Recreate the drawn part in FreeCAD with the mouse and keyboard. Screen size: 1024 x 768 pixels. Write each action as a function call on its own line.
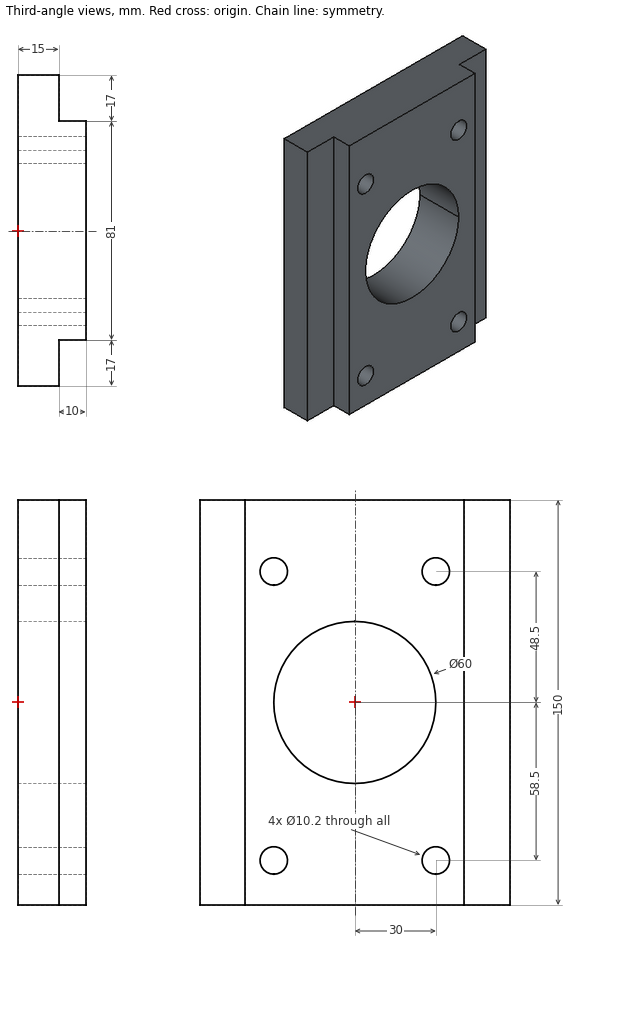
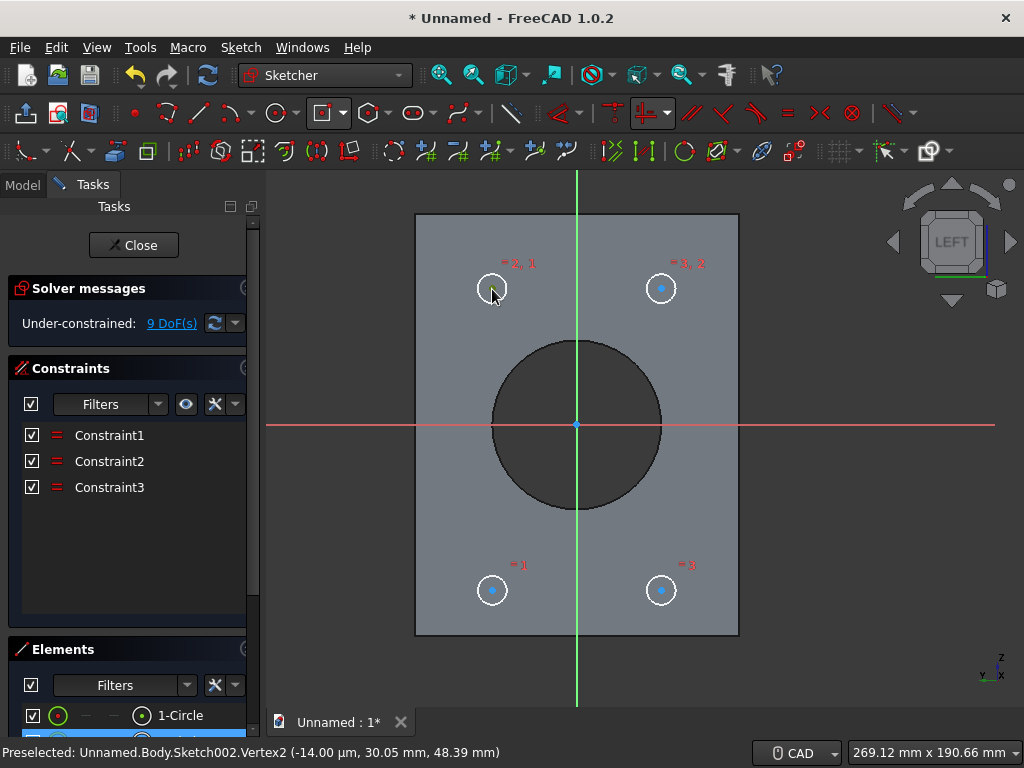
click(661, 289)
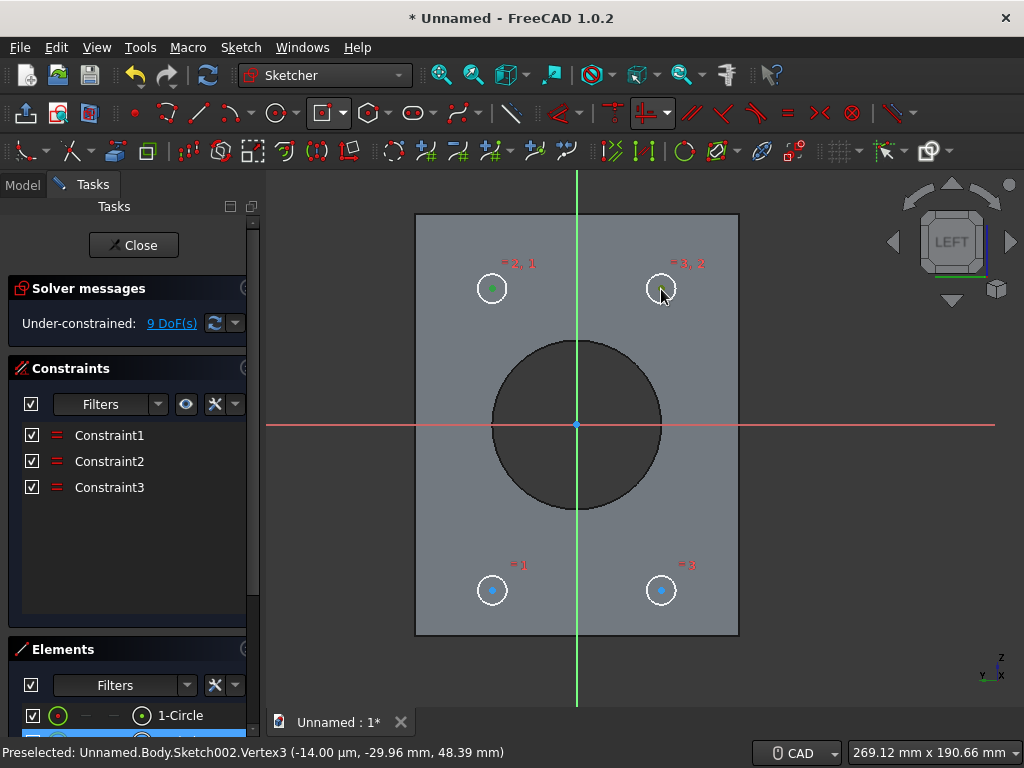
click(577, 645)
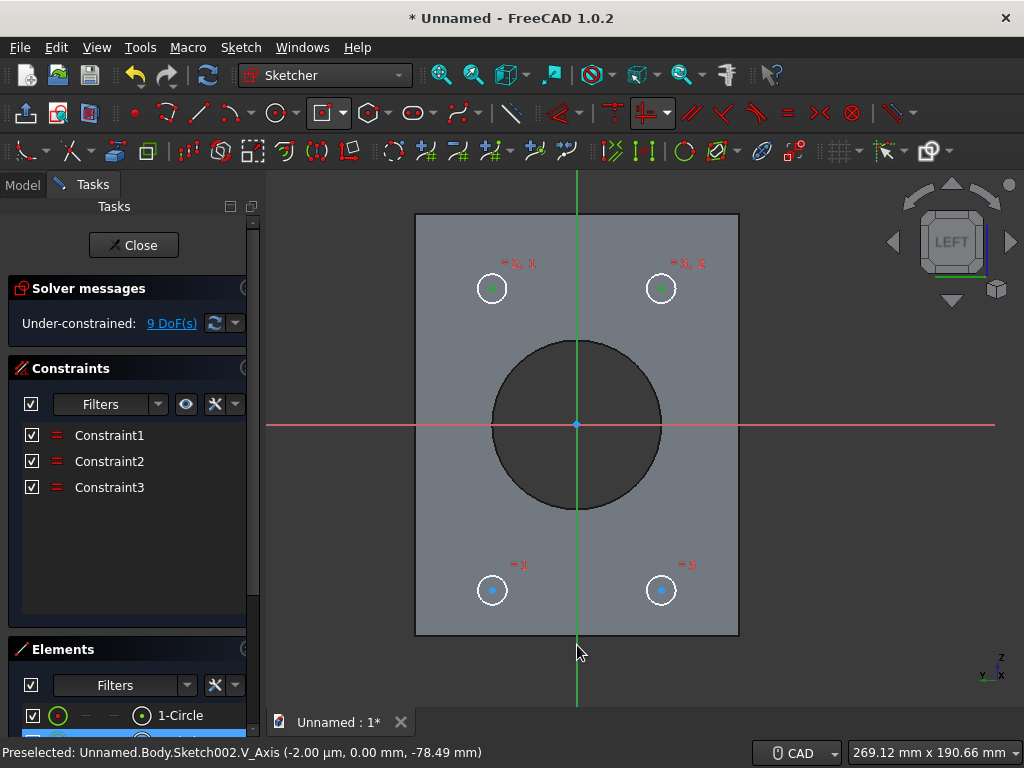
click(820, 114)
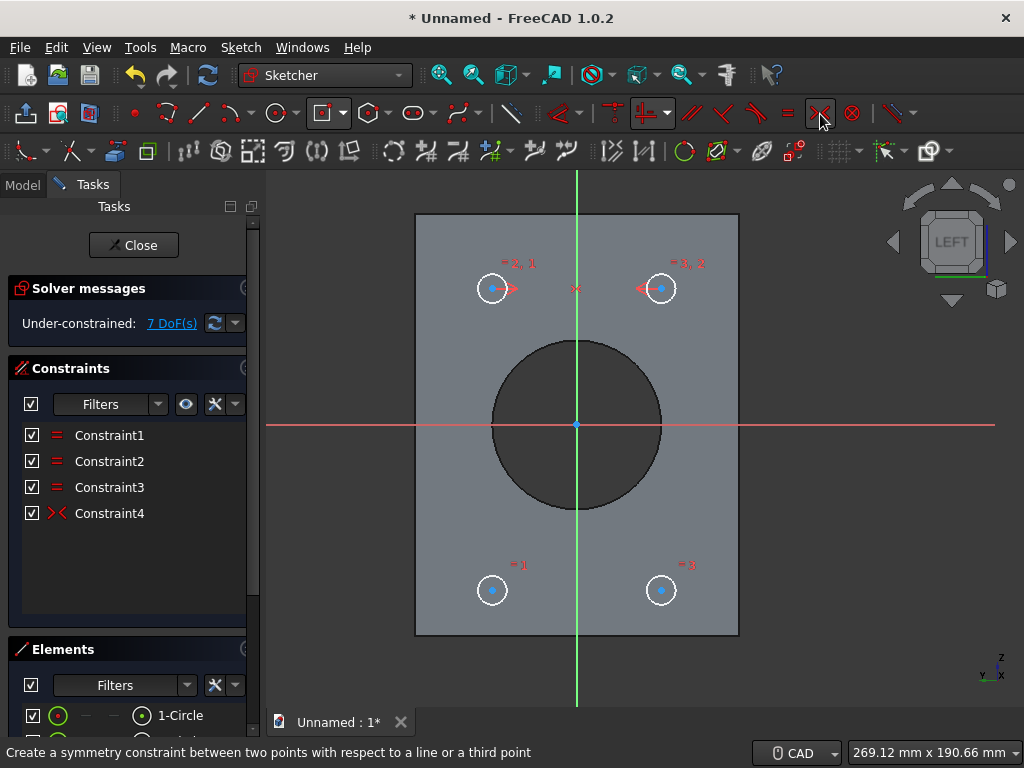
click(492, 590)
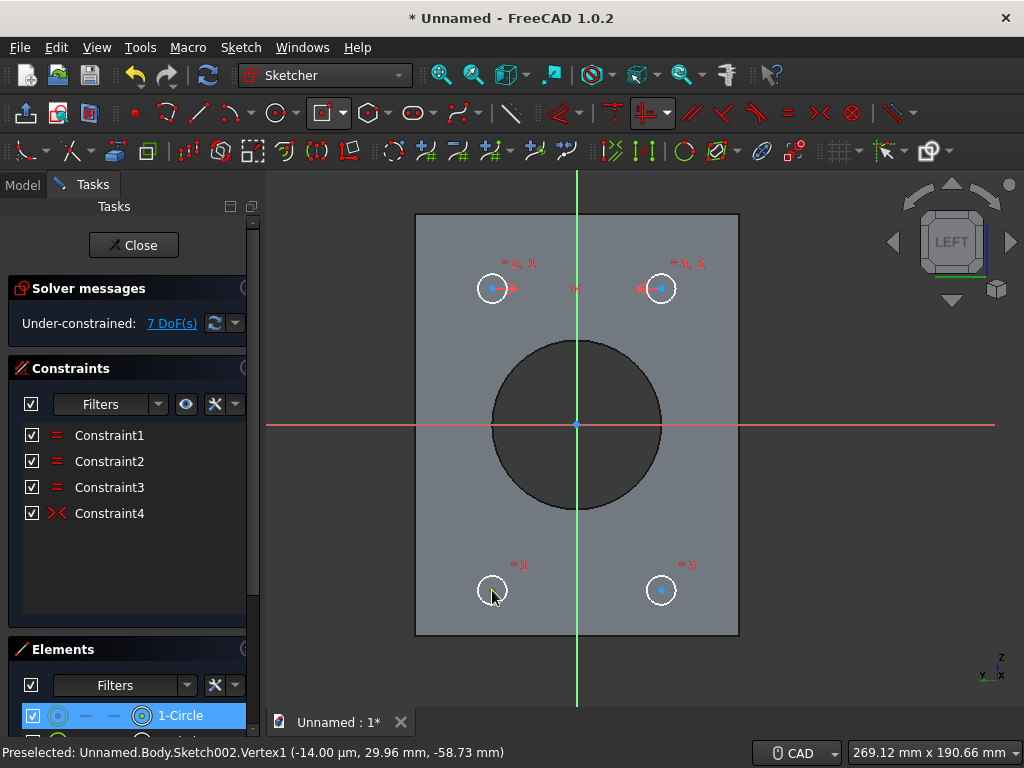
click(661, 590)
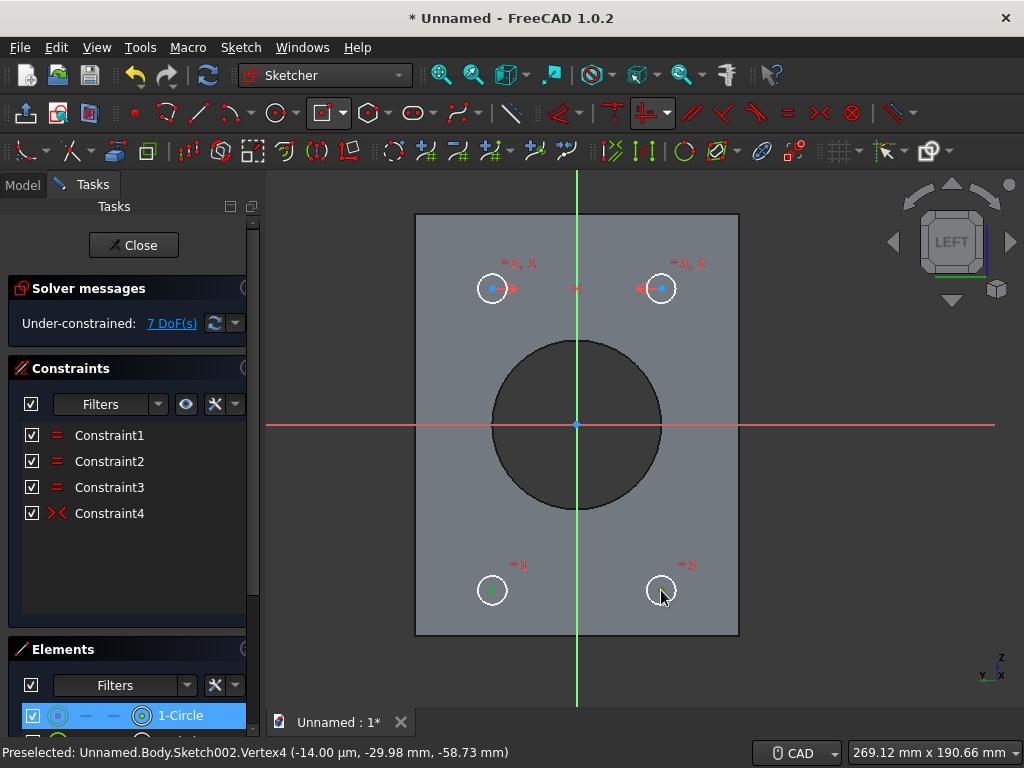
click(577, 645)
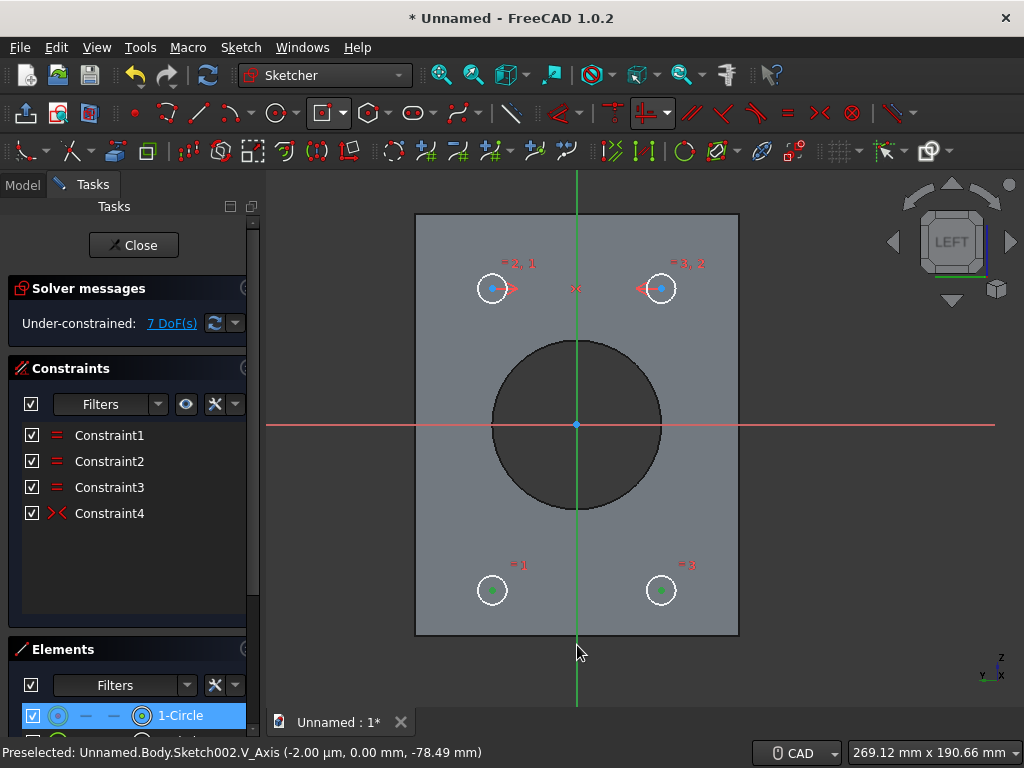
click(820, 114)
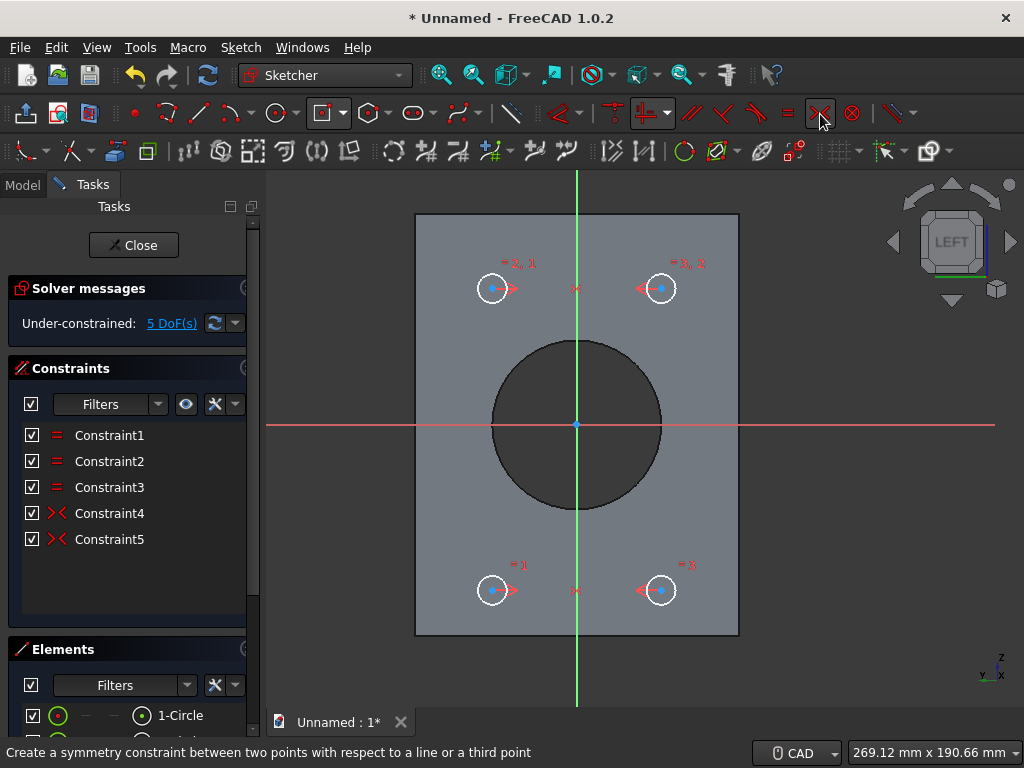
click(558, 114)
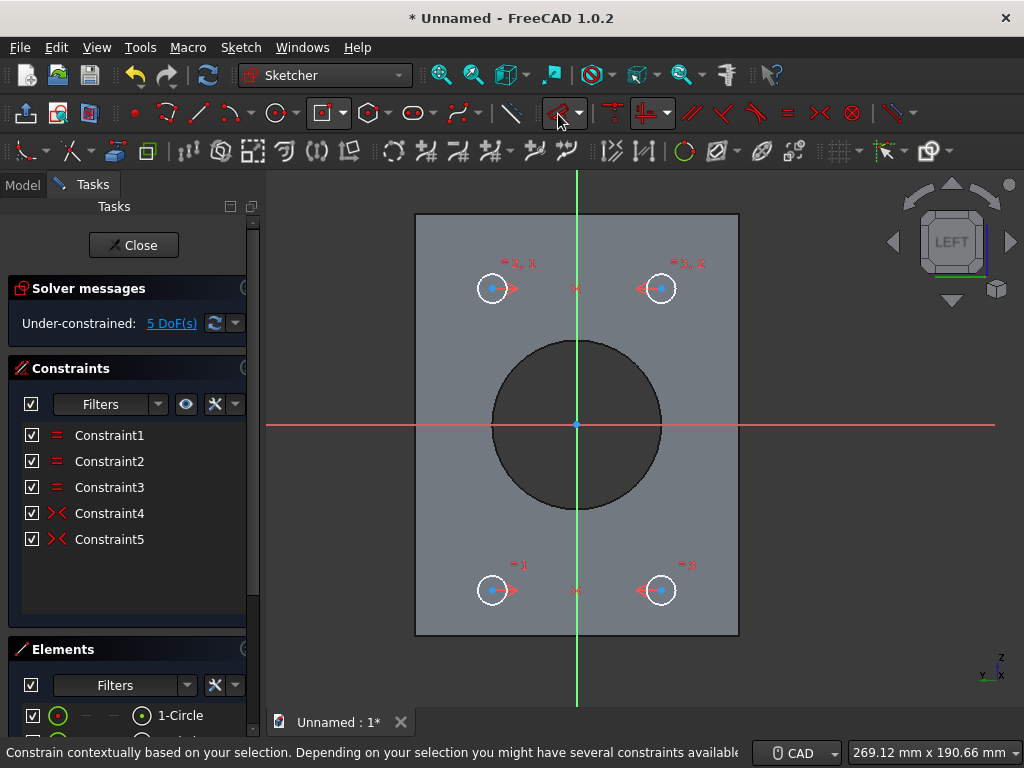
scroll(503, 580, up, 2)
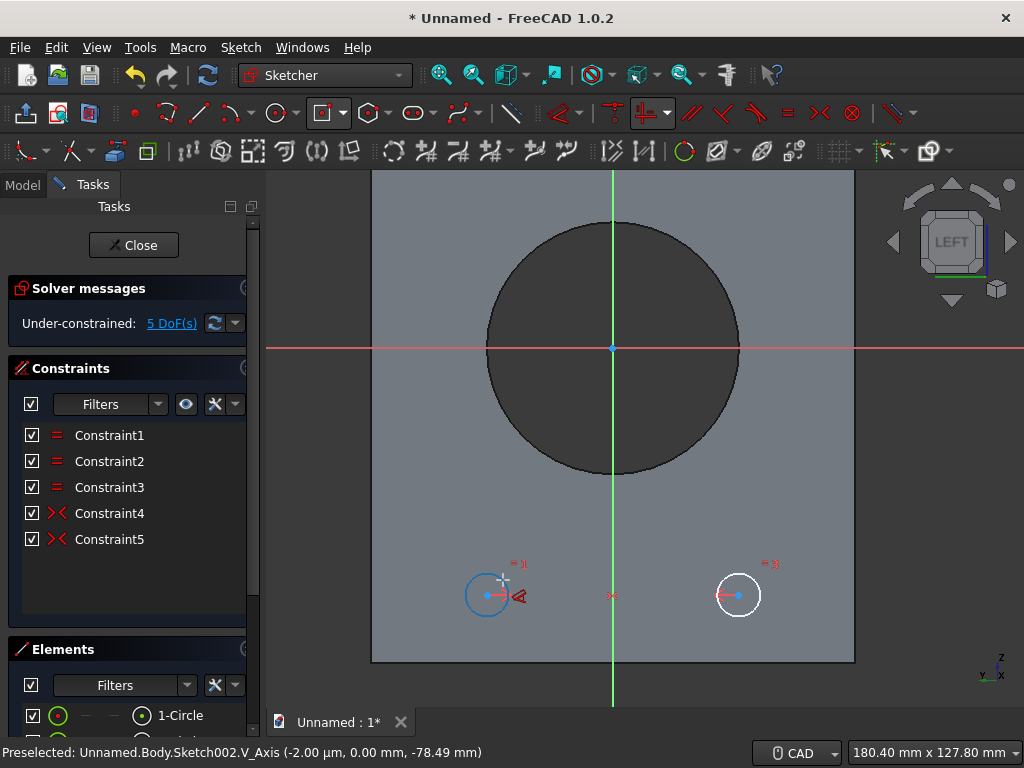
click(502, 580)
click(525, 557)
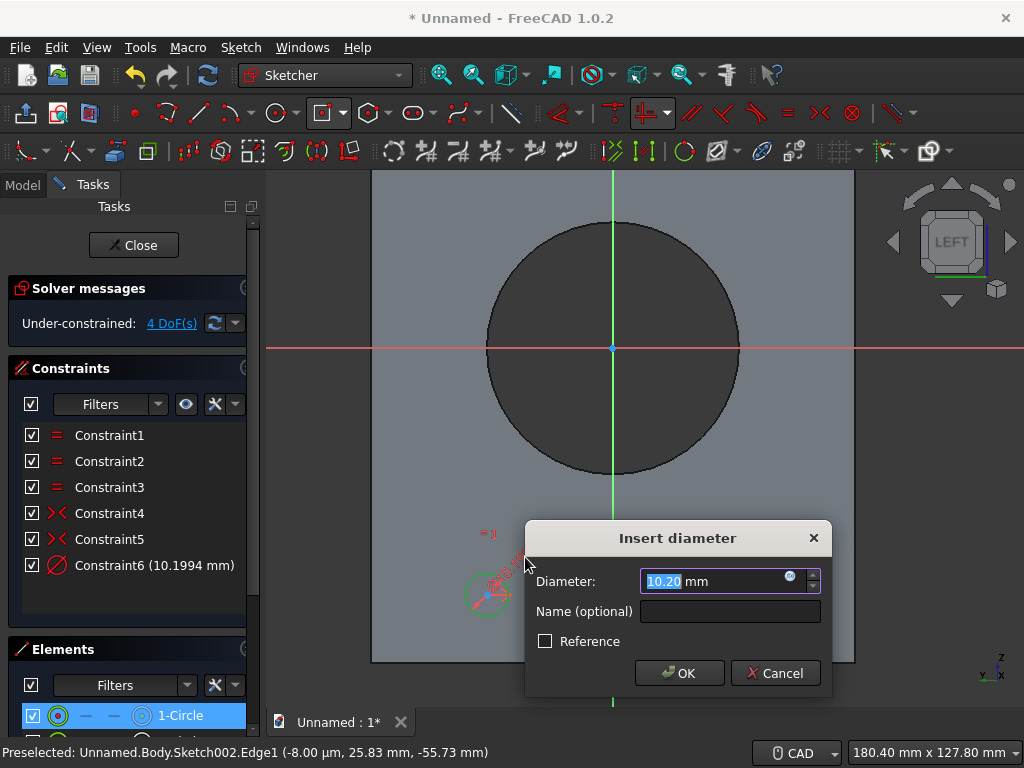
text(10.2)
key(Return)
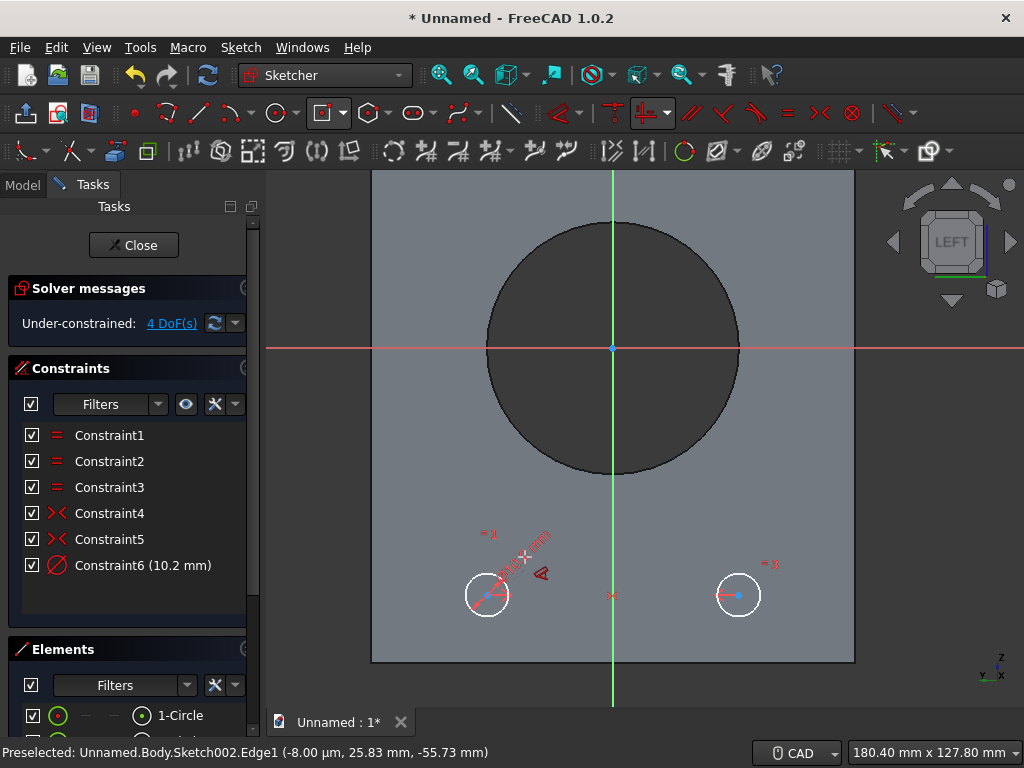
click(487, 595)
click(550, 629)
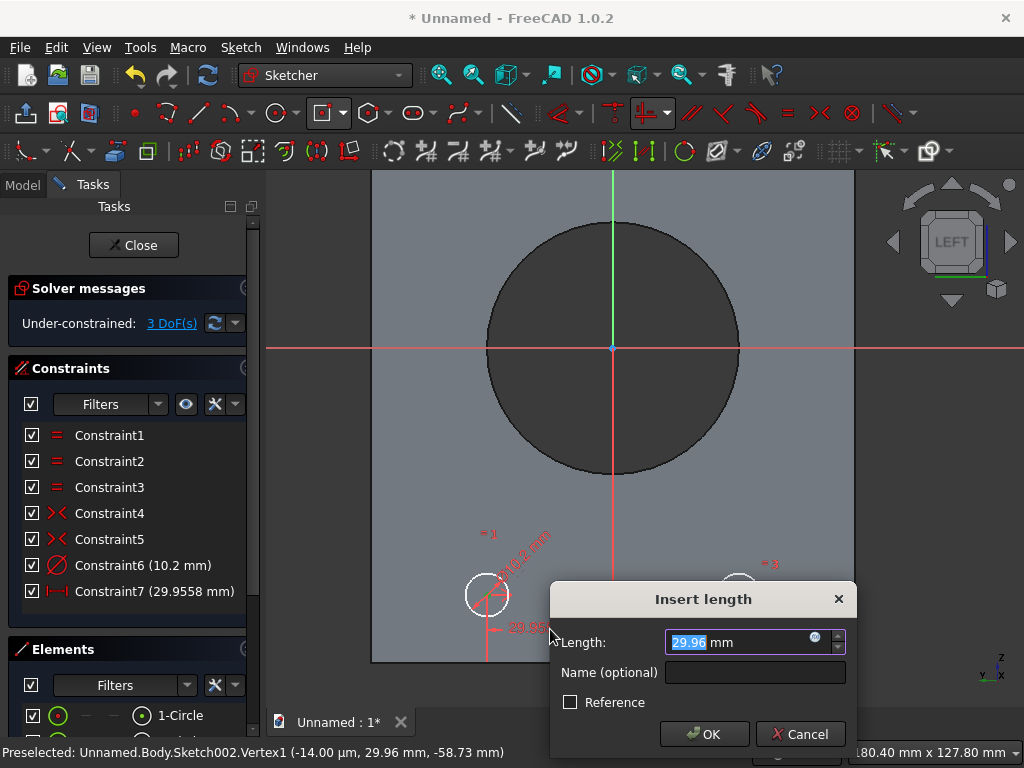
text(30)
key(Return)